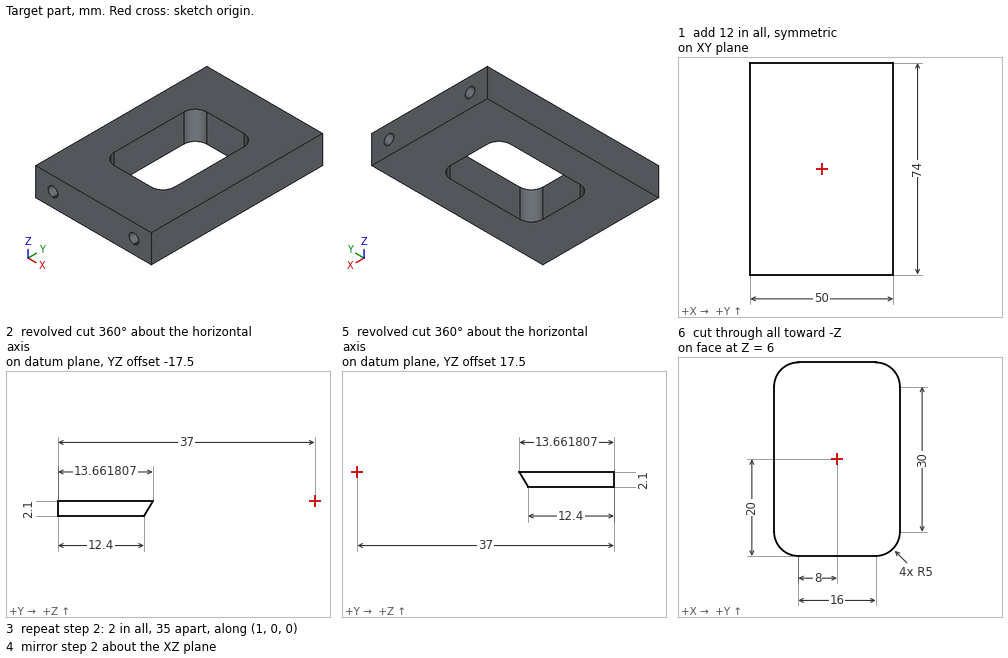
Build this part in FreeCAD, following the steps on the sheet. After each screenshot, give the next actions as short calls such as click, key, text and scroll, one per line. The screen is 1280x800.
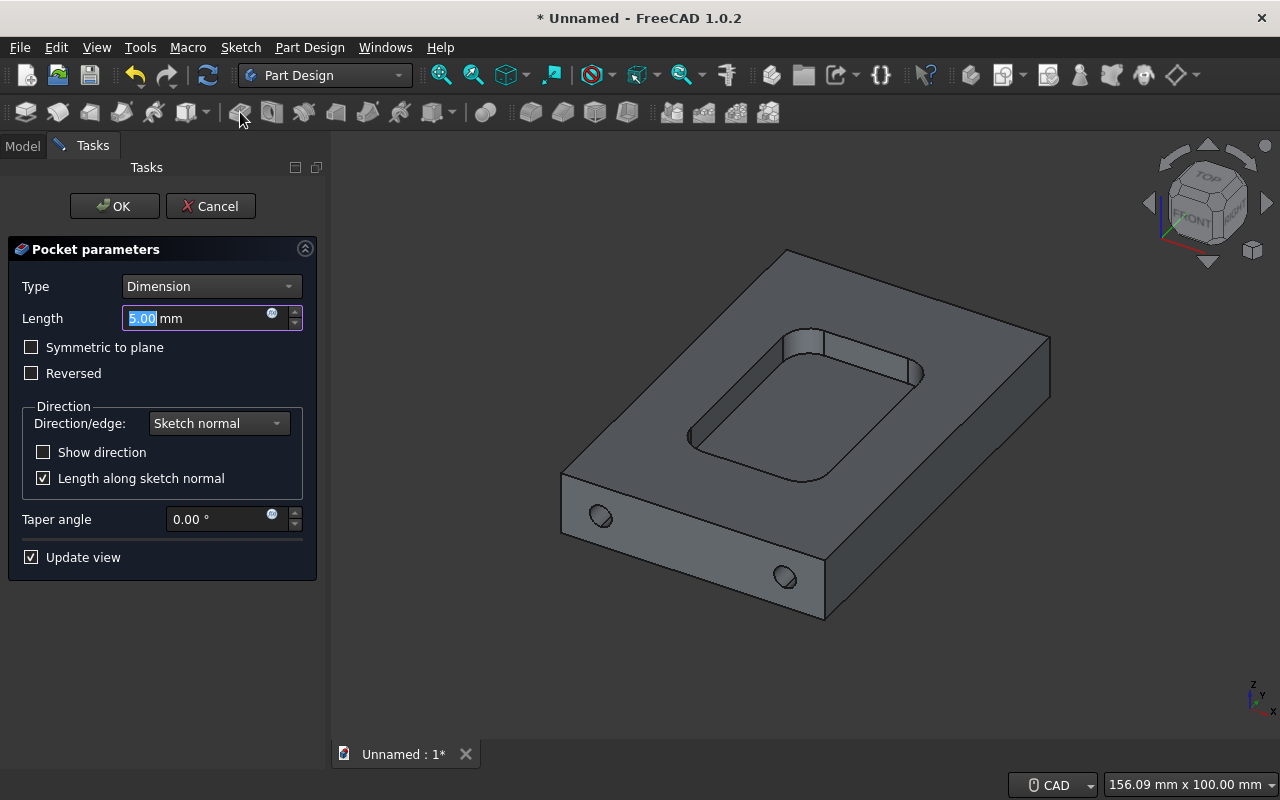
click(212, 286)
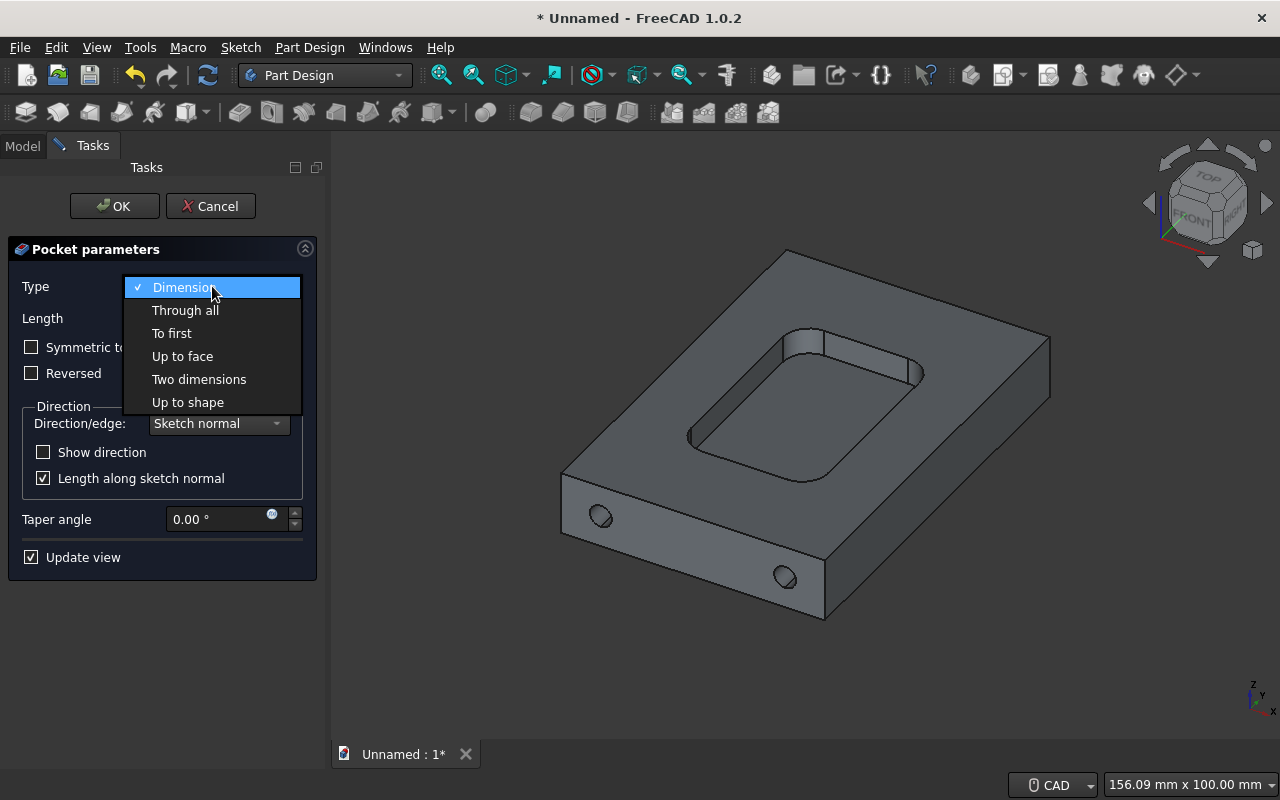
click(212, 310)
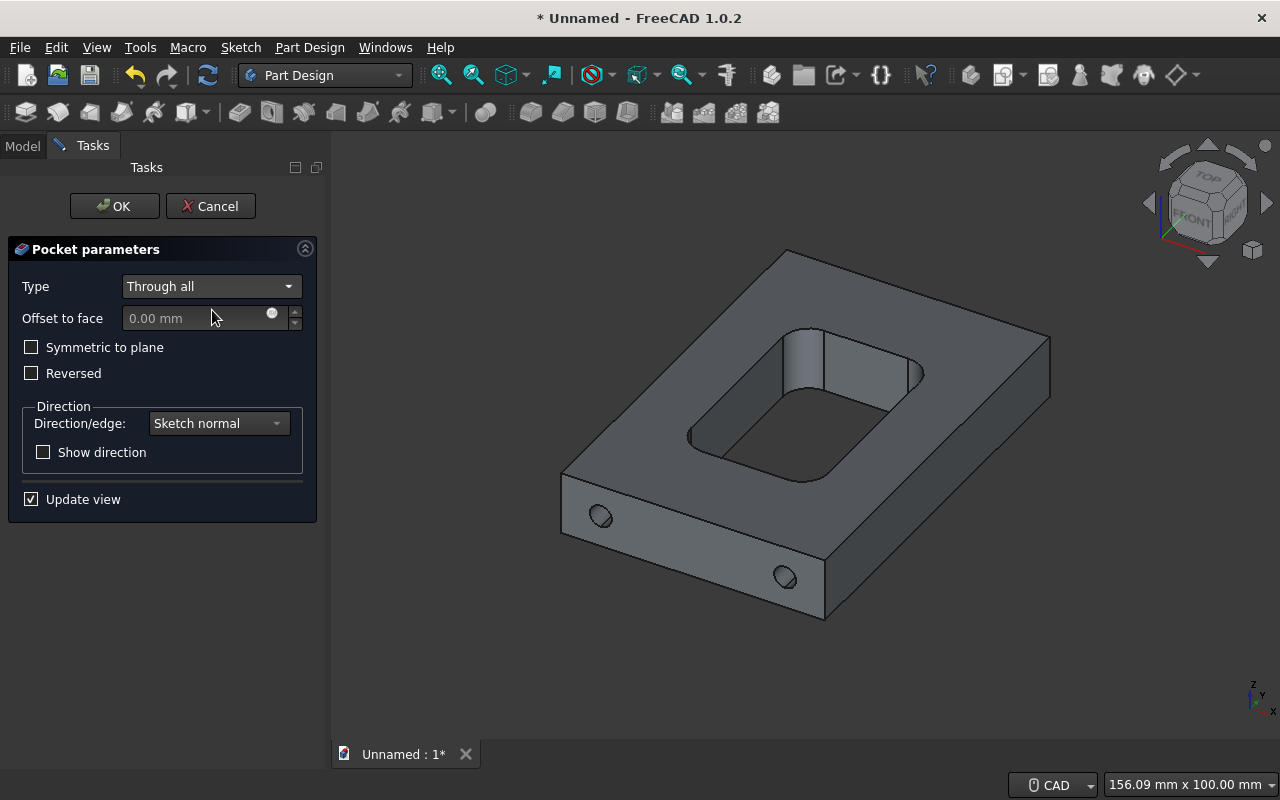
click(115, 206)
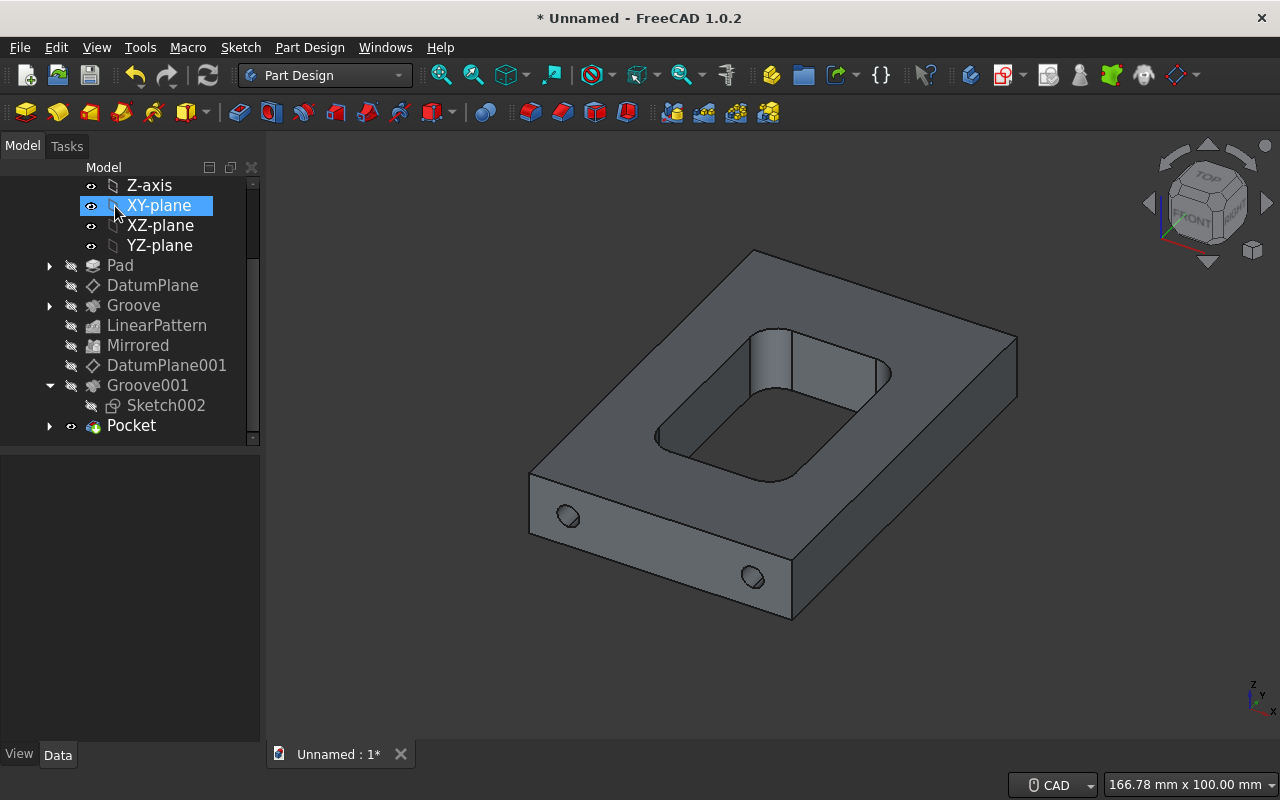
key(0)